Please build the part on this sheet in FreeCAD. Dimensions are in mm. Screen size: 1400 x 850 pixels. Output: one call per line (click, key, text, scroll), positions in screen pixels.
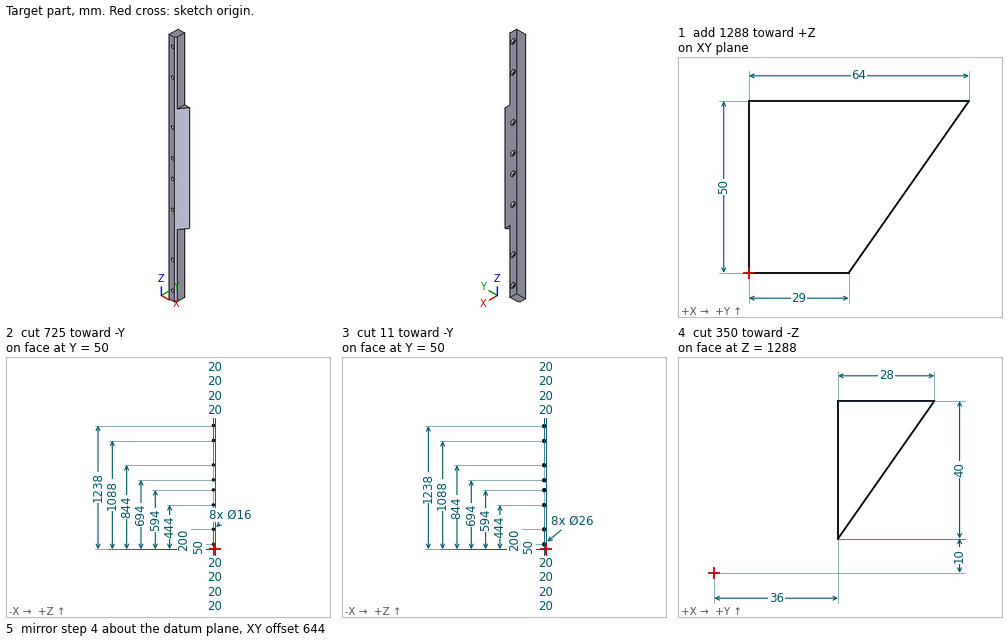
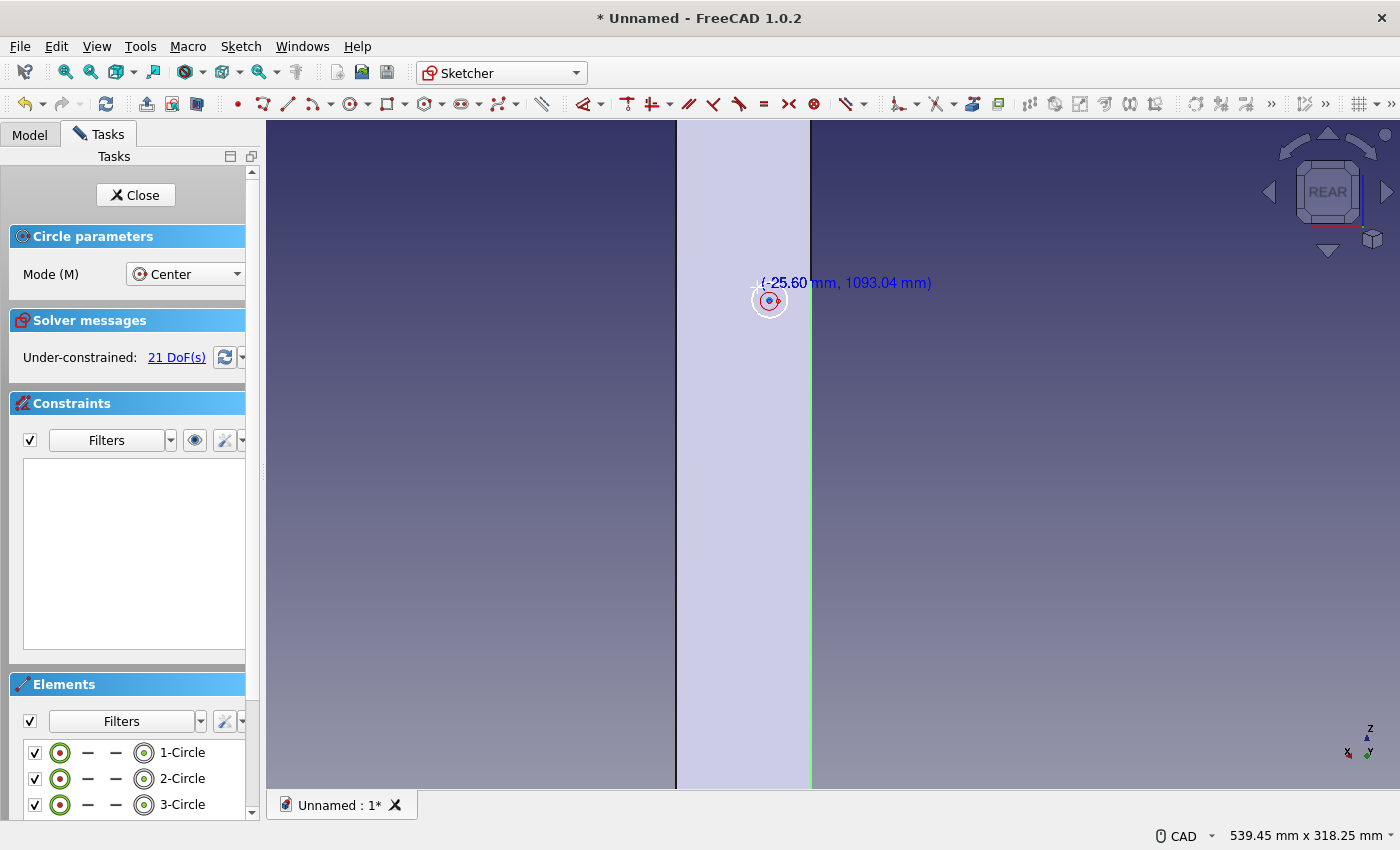
scroll(761, 292, down, 9)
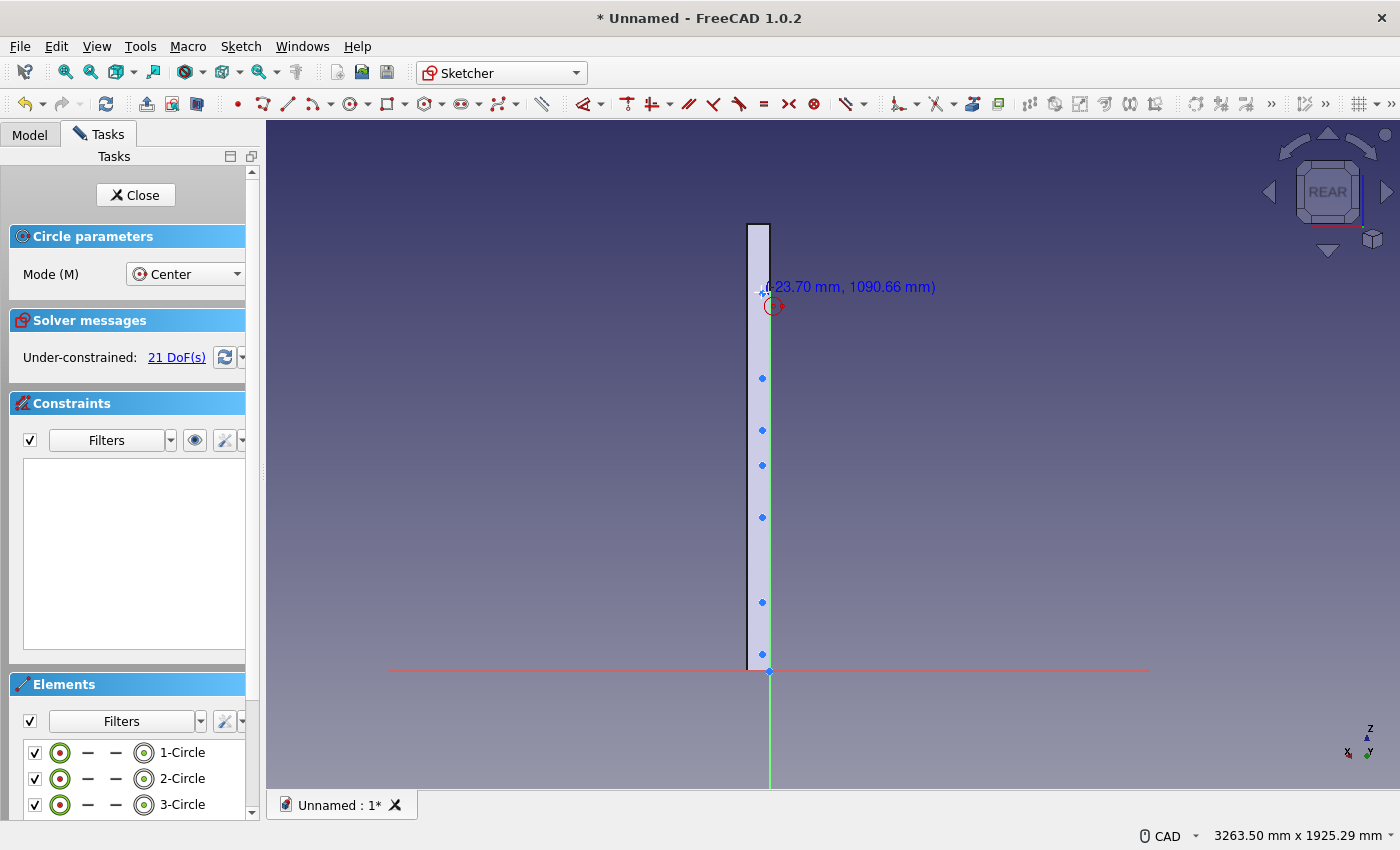
scroll(763, 241, up, 11)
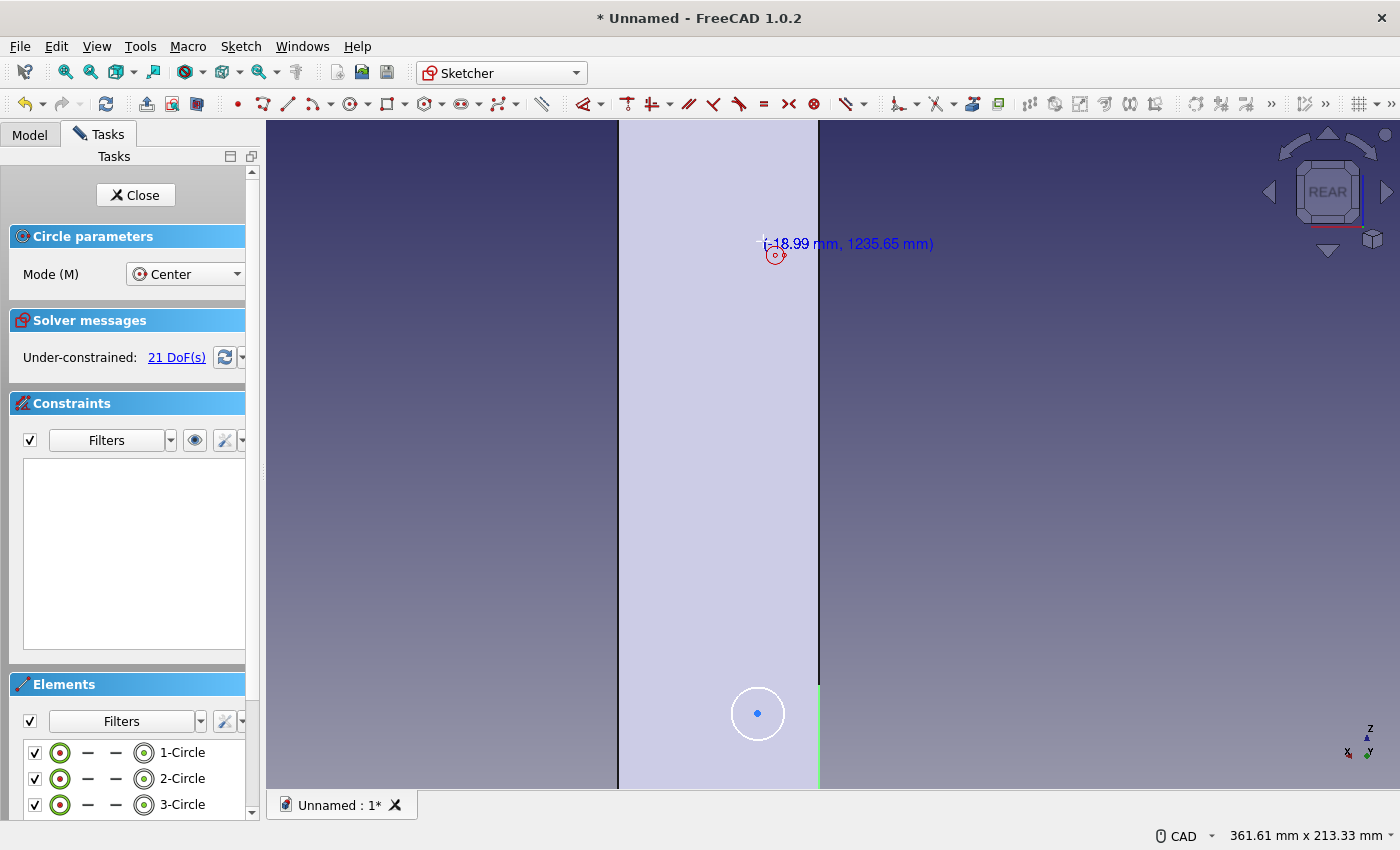
scroll(763, 241, down, 11)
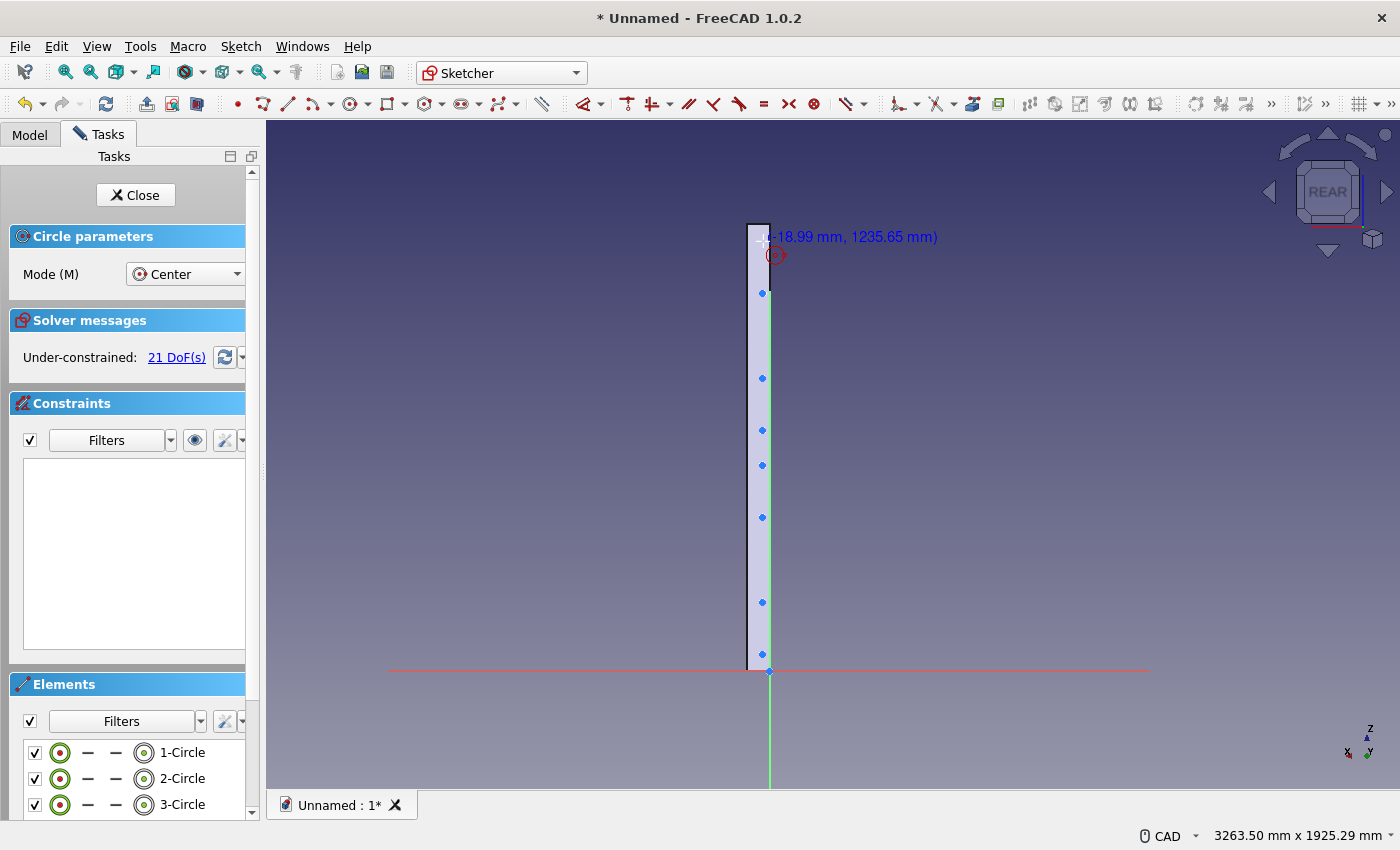
scroll(763, 241, up, 5)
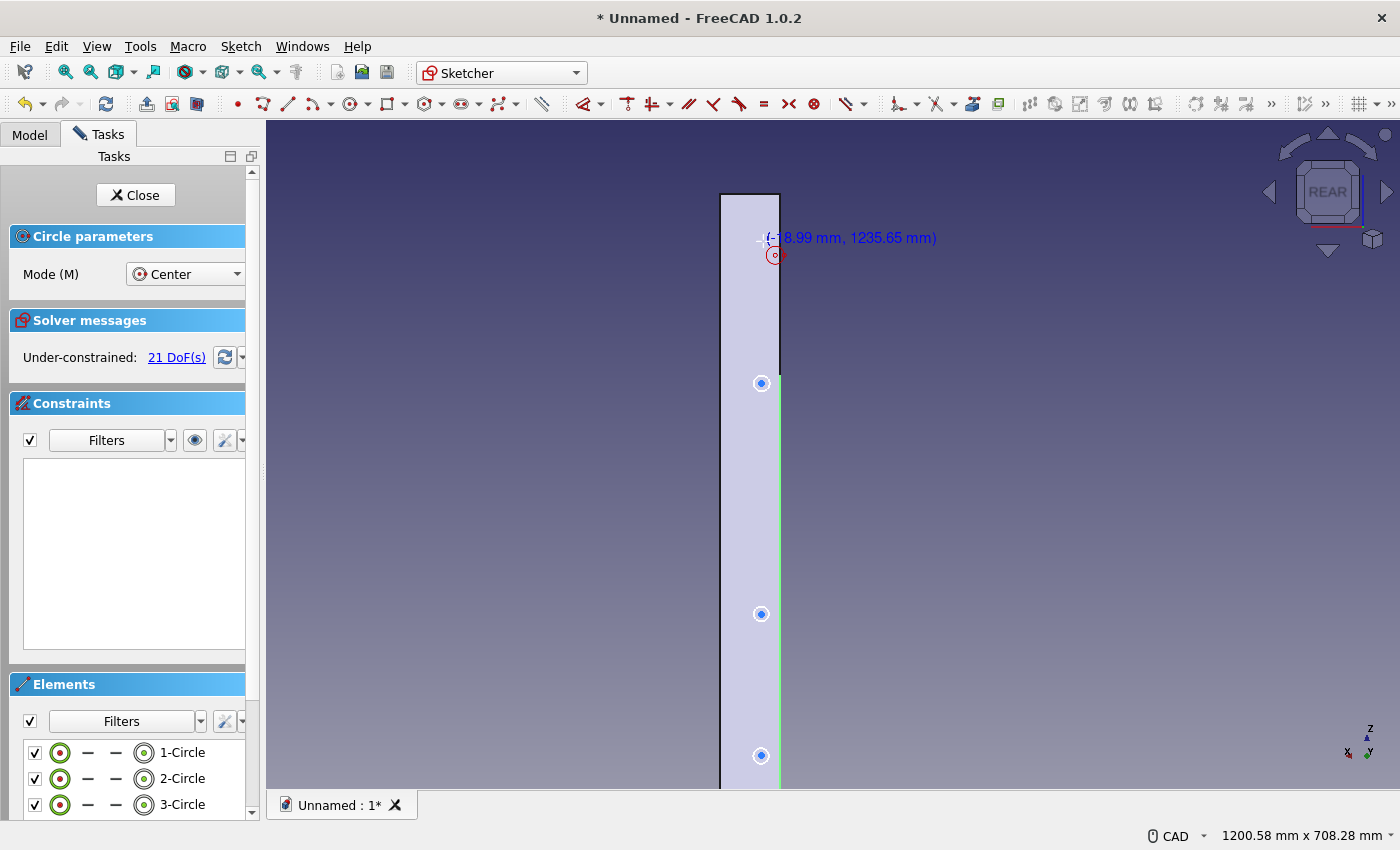
click(761, 241)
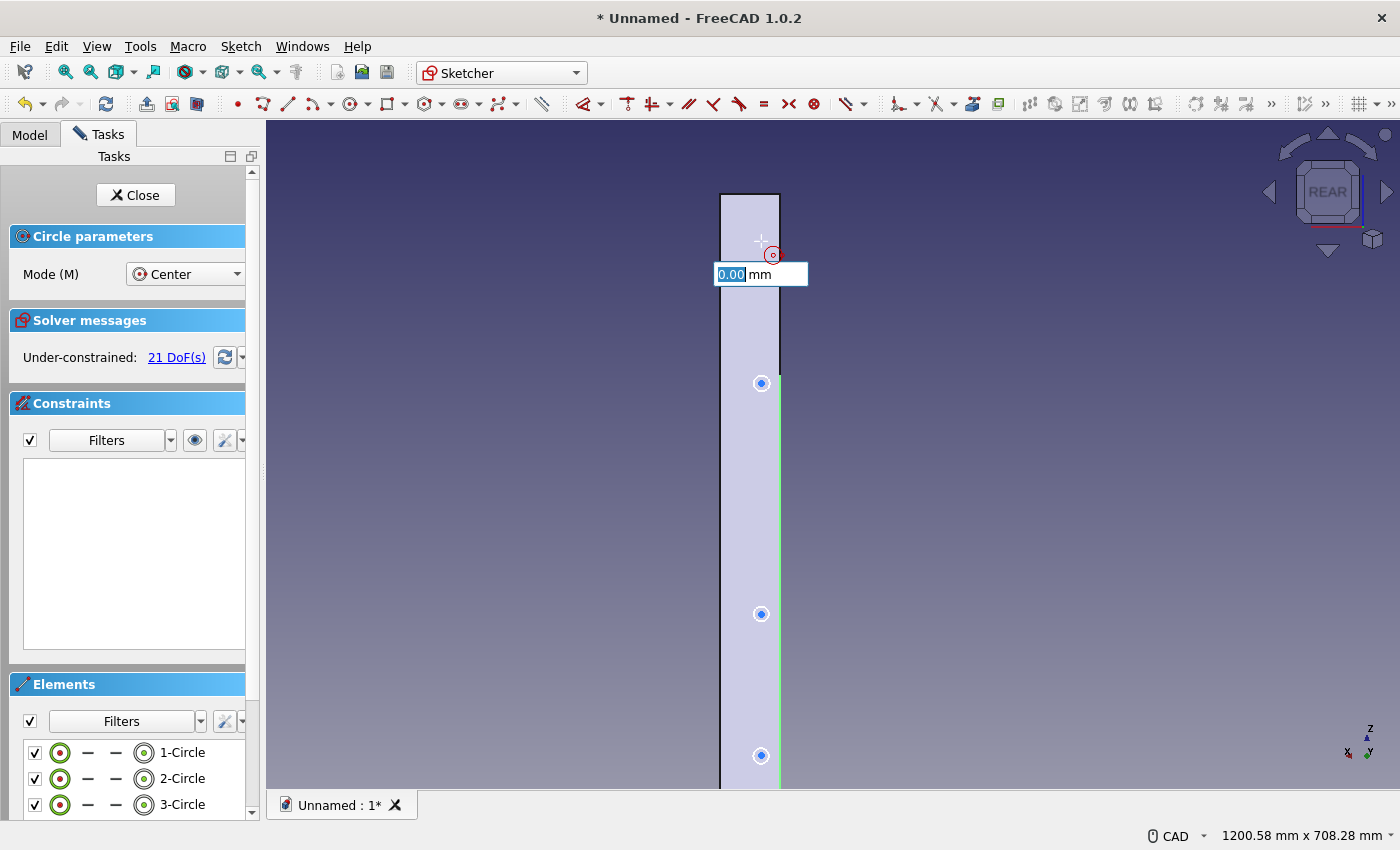
scroll(756, 236, up, 4)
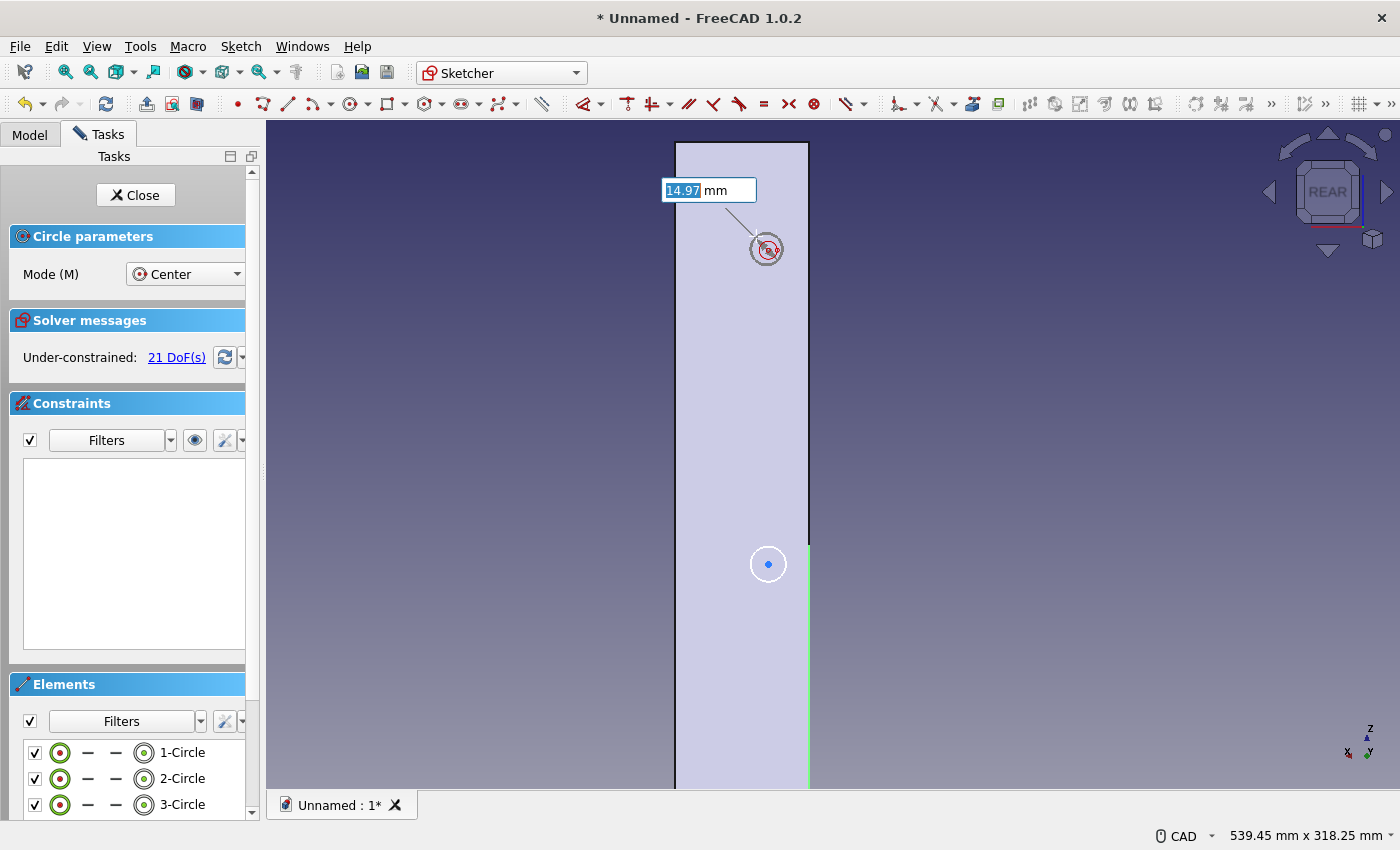
click(755, 235)
key(Escape)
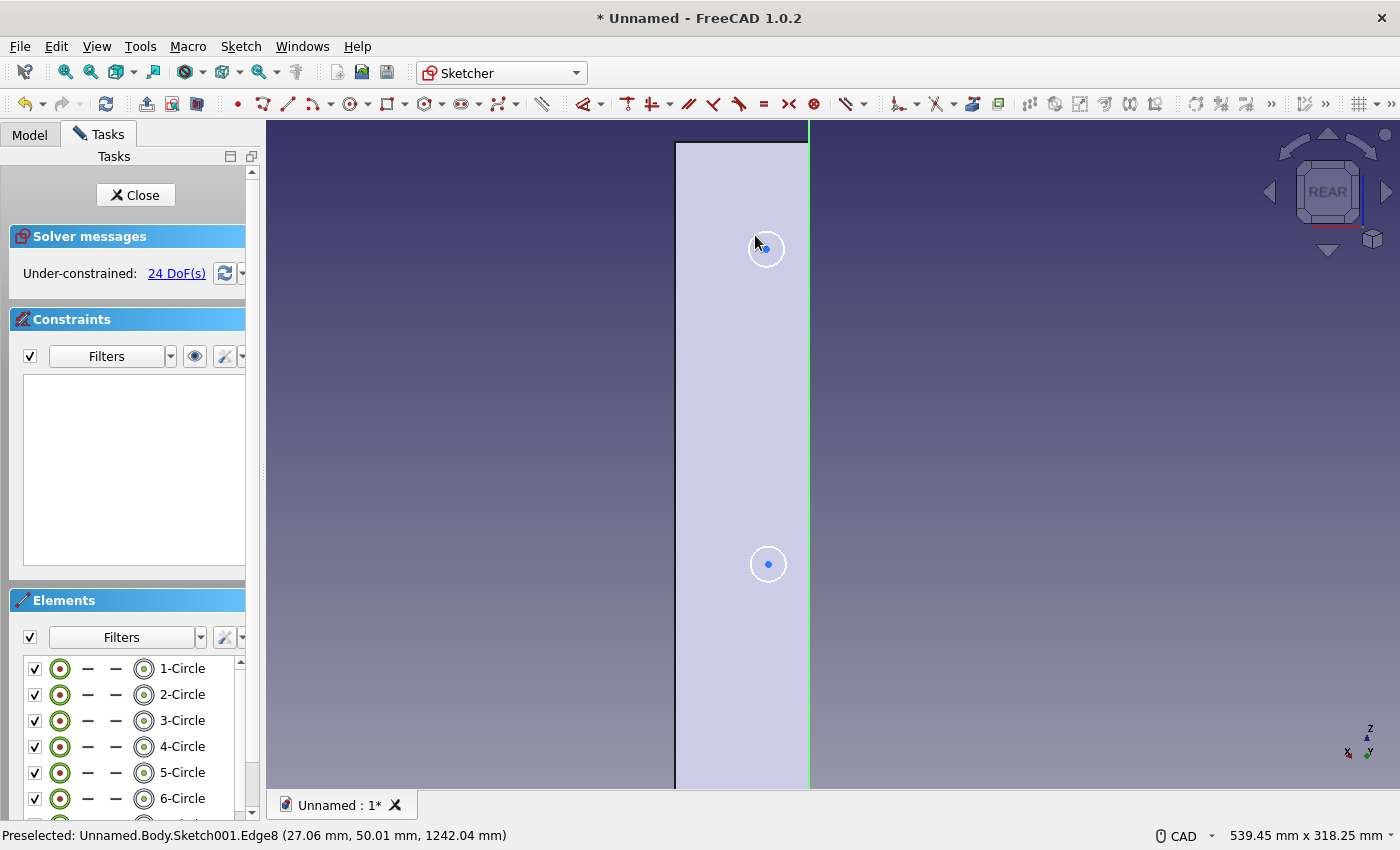
scroll(761, 240, down, 9)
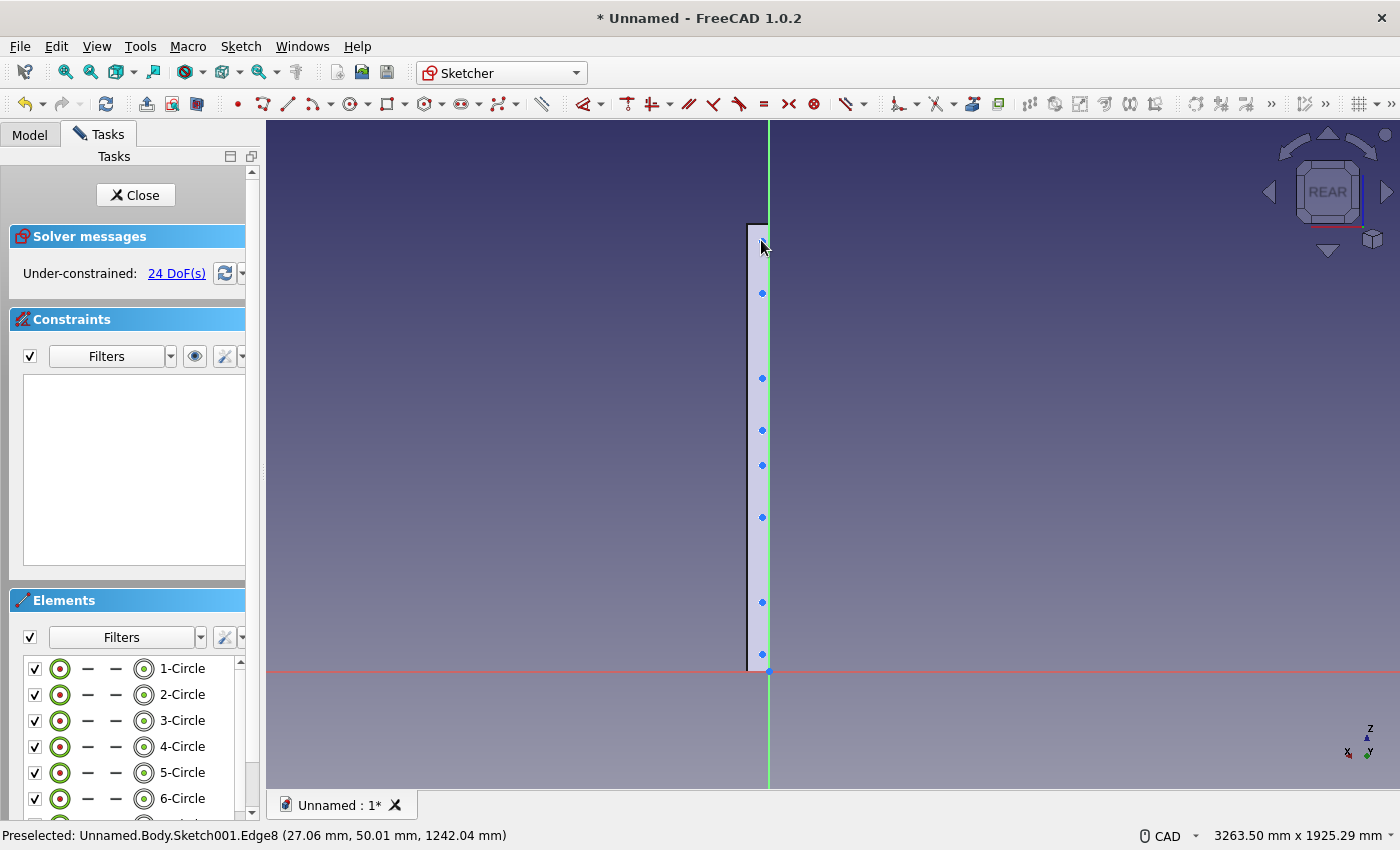
scroll(764, 652, up, 9)